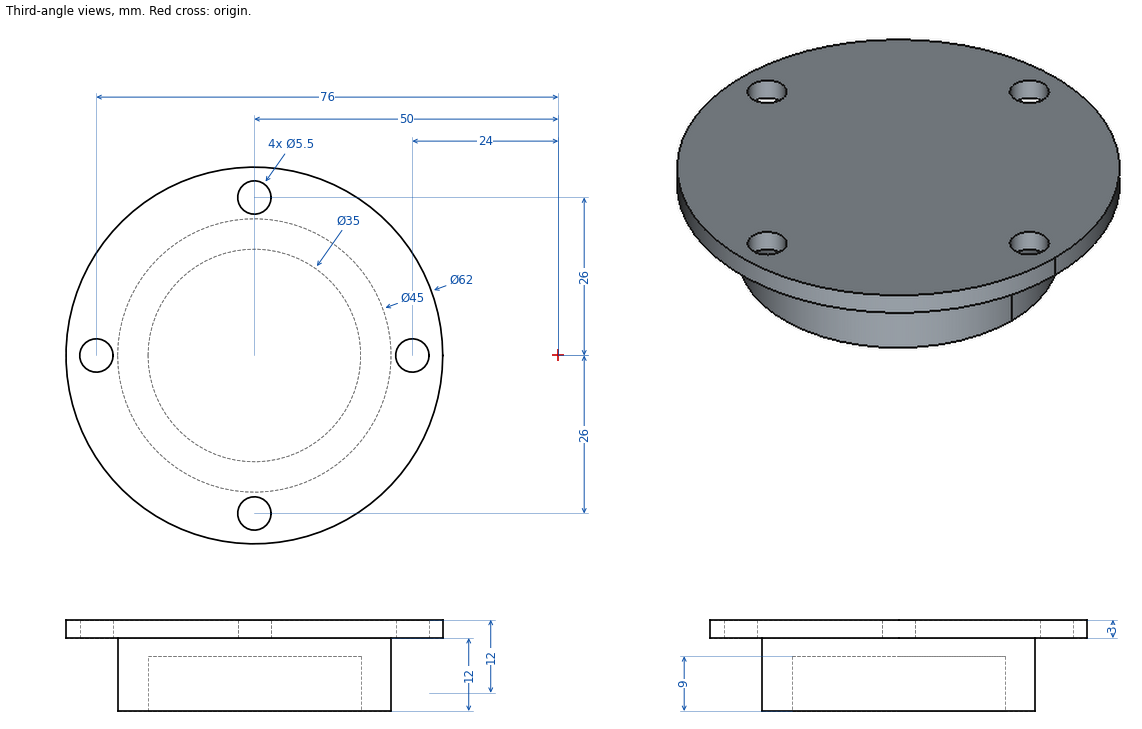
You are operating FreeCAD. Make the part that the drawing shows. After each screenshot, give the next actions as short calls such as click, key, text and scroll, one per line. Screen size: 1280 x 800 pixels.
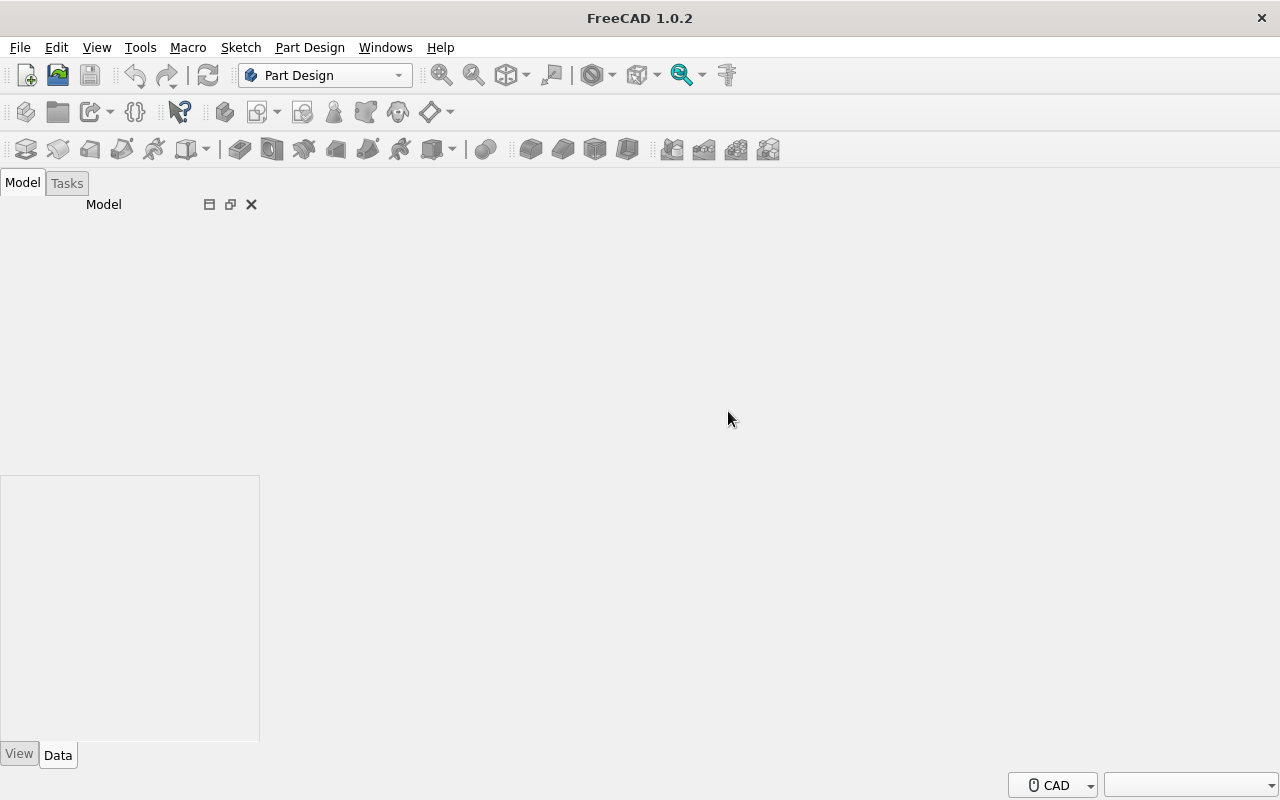
click(26, 76)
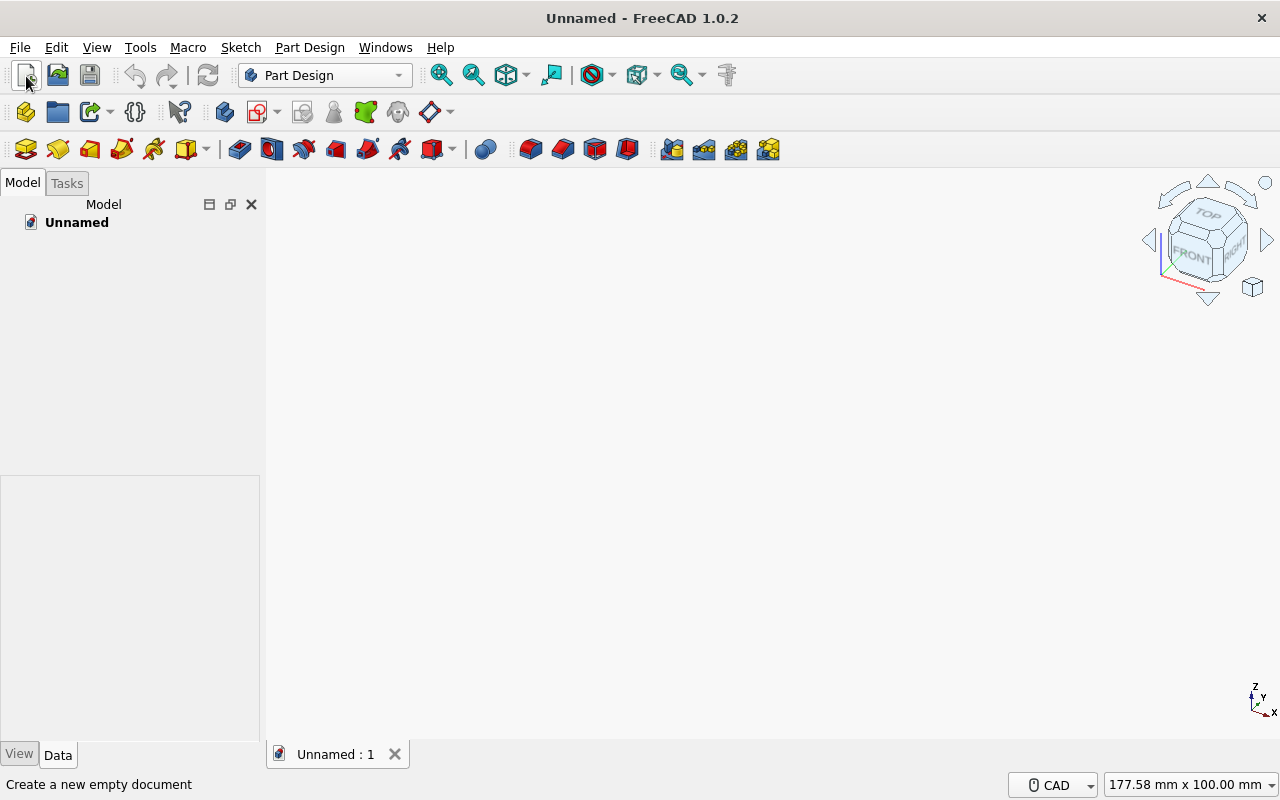
click(226, 112)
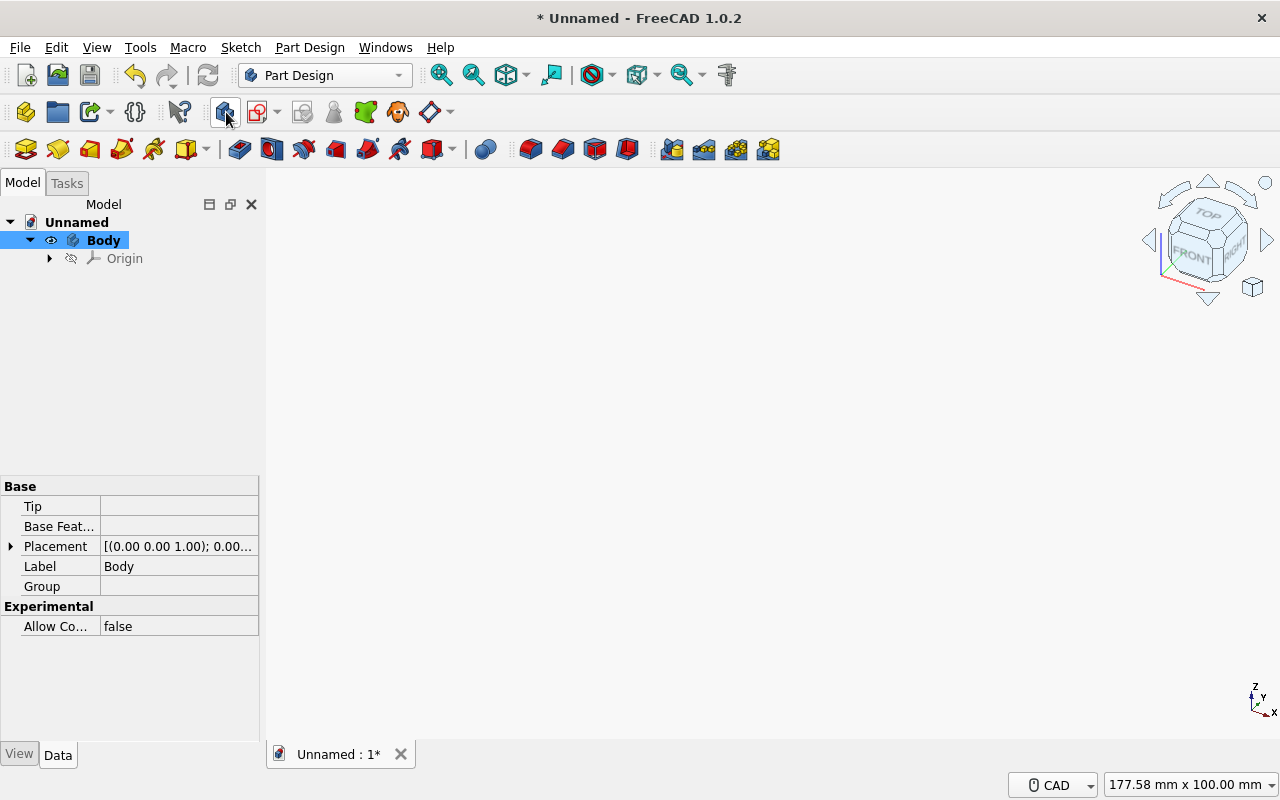
click(50, 258)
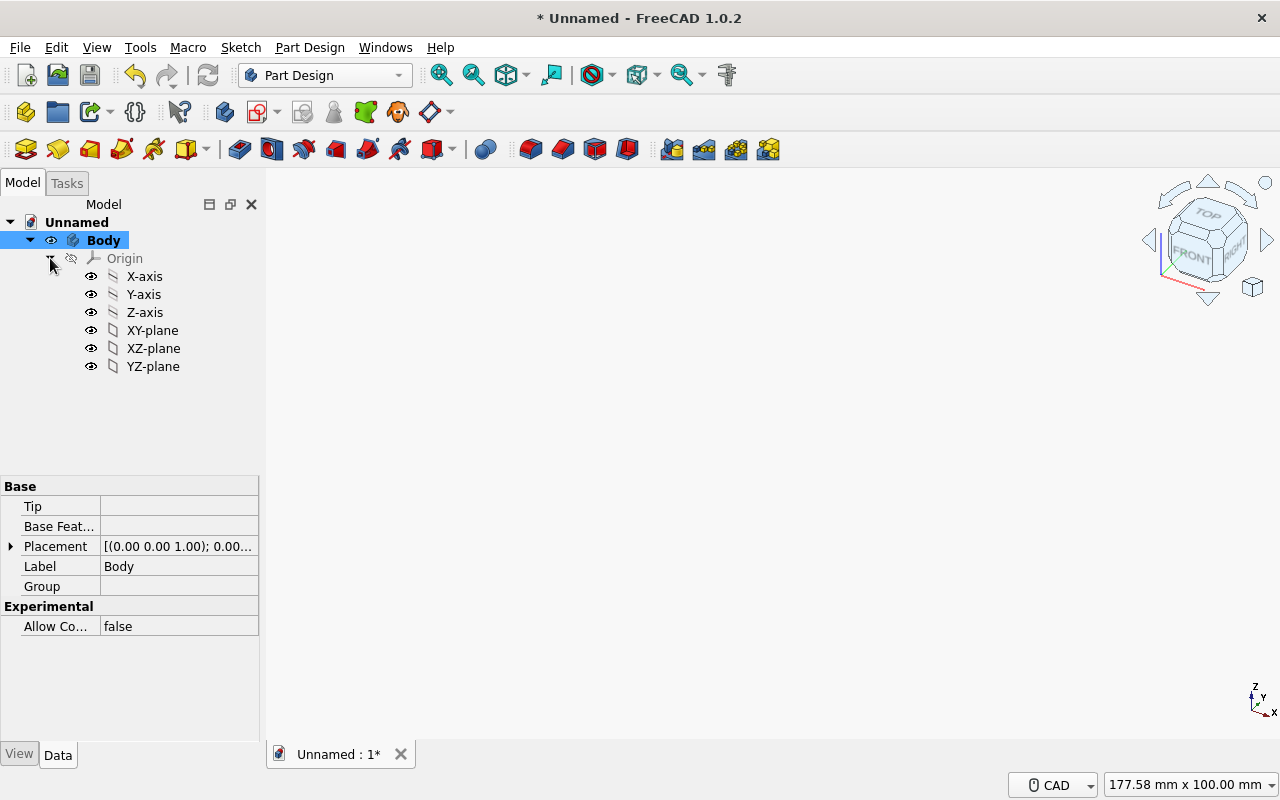
click(136, 330)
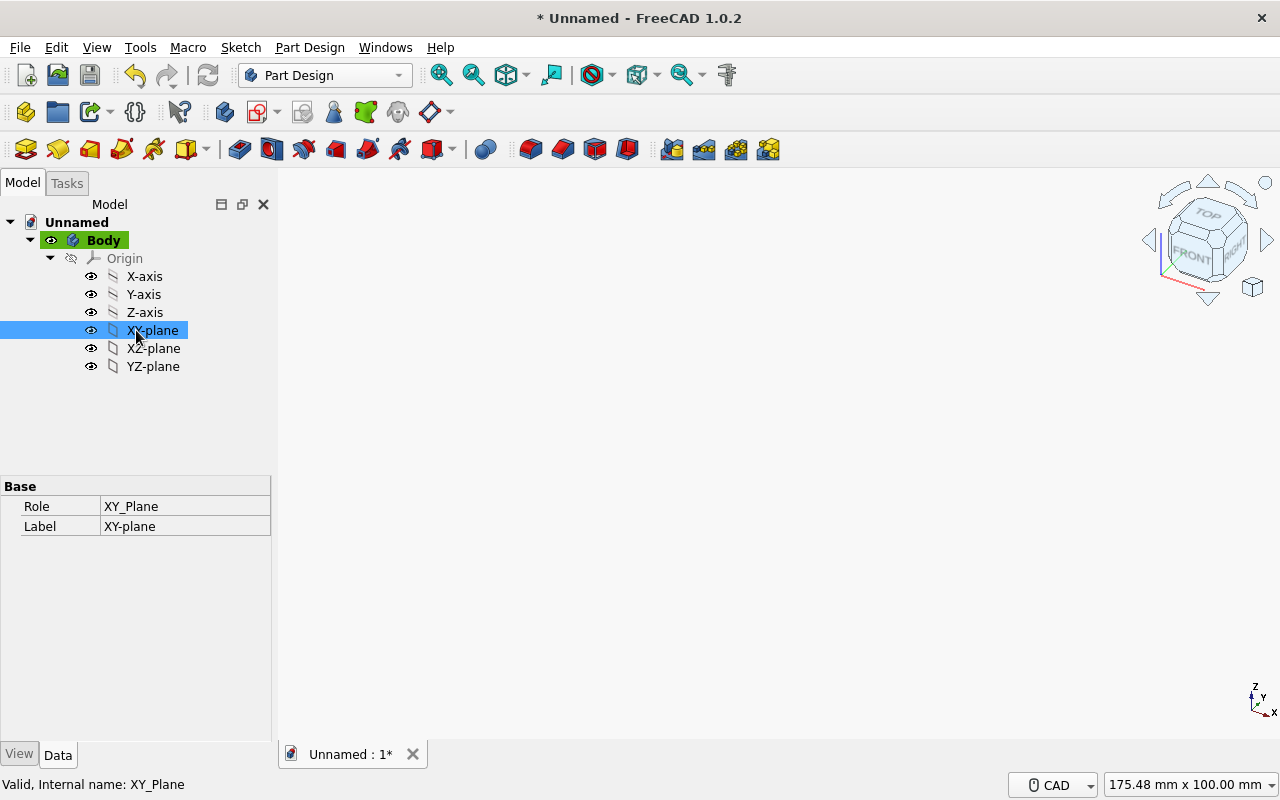
click(430, 112)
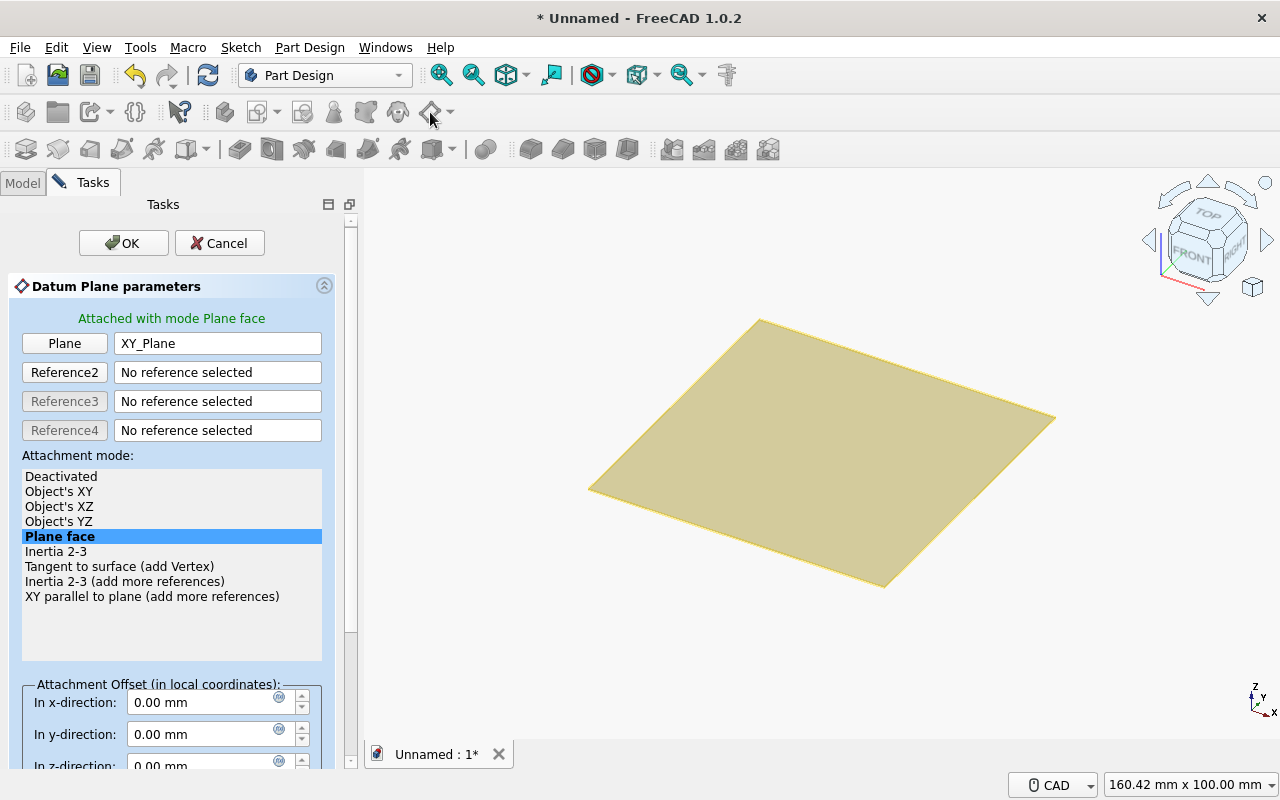
scroll(351, 491, down, 2)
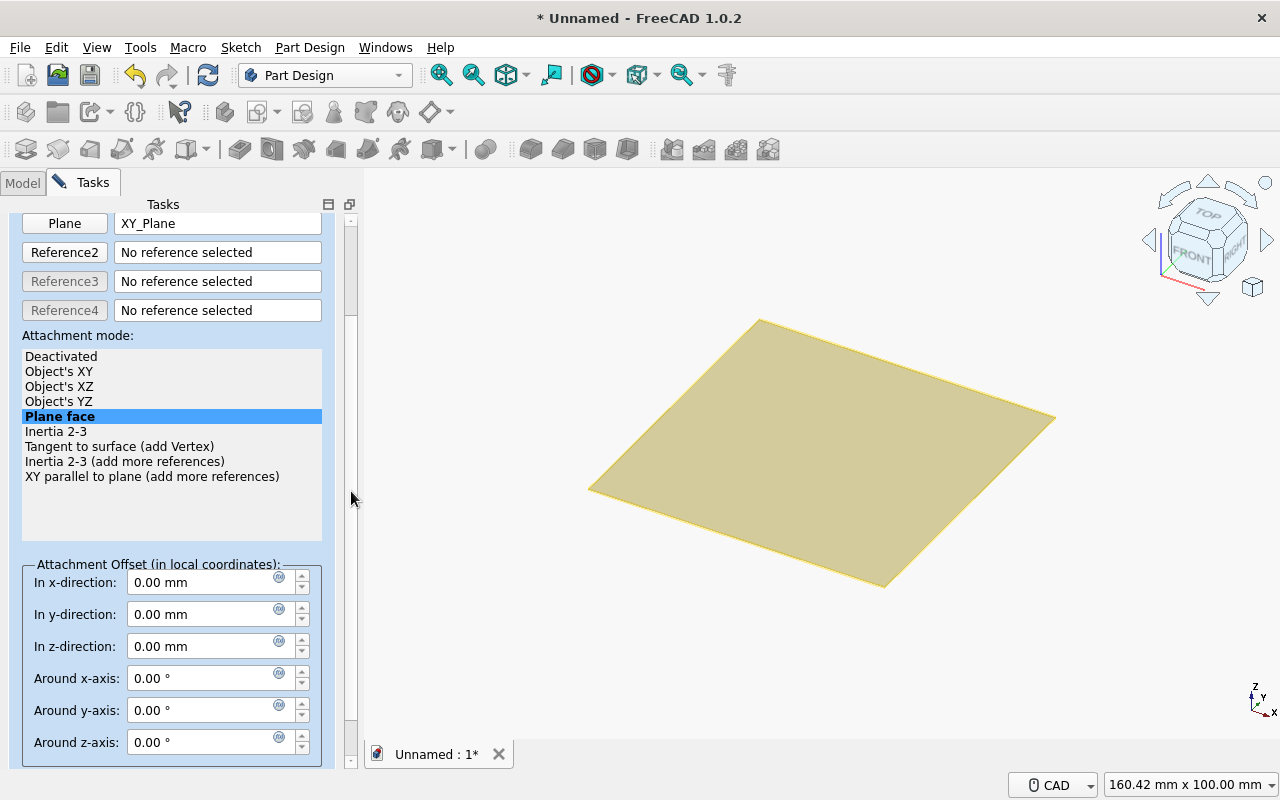
triple_click(210, 646)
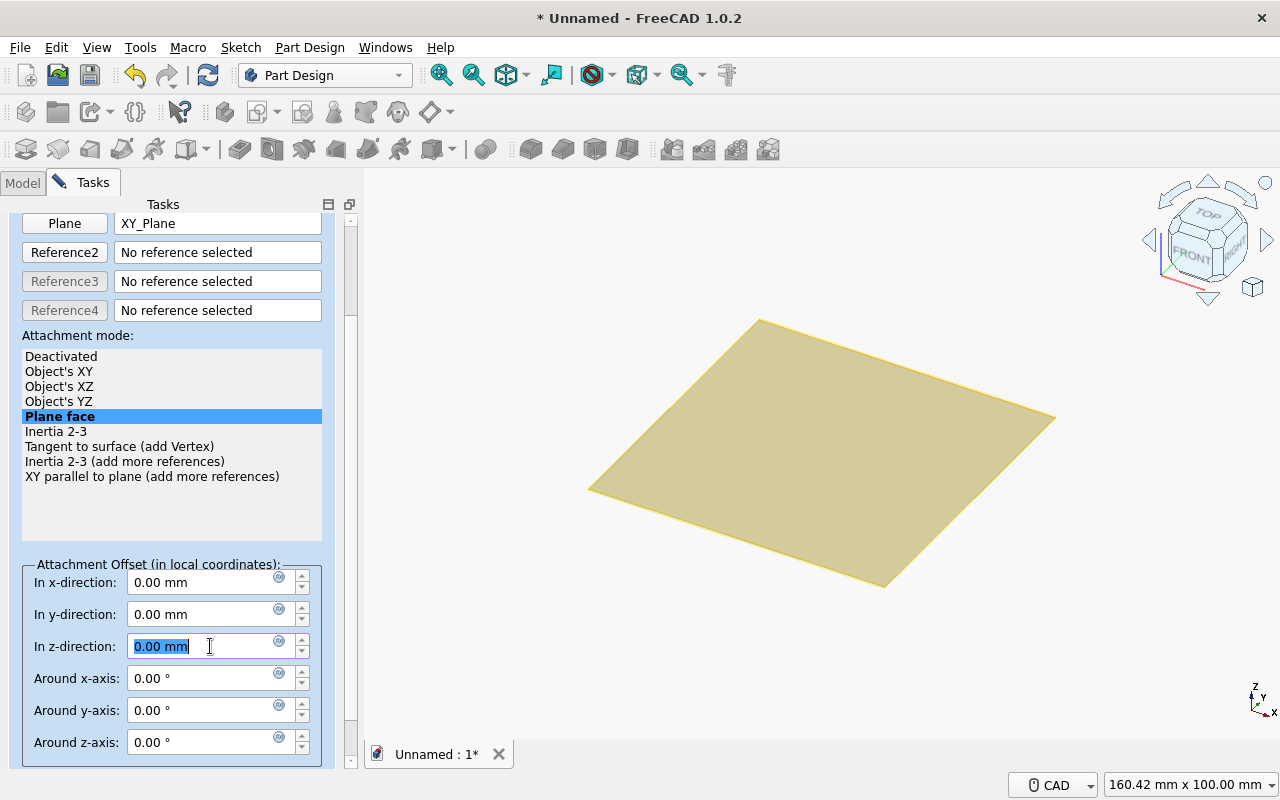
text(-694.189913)
key(Tab)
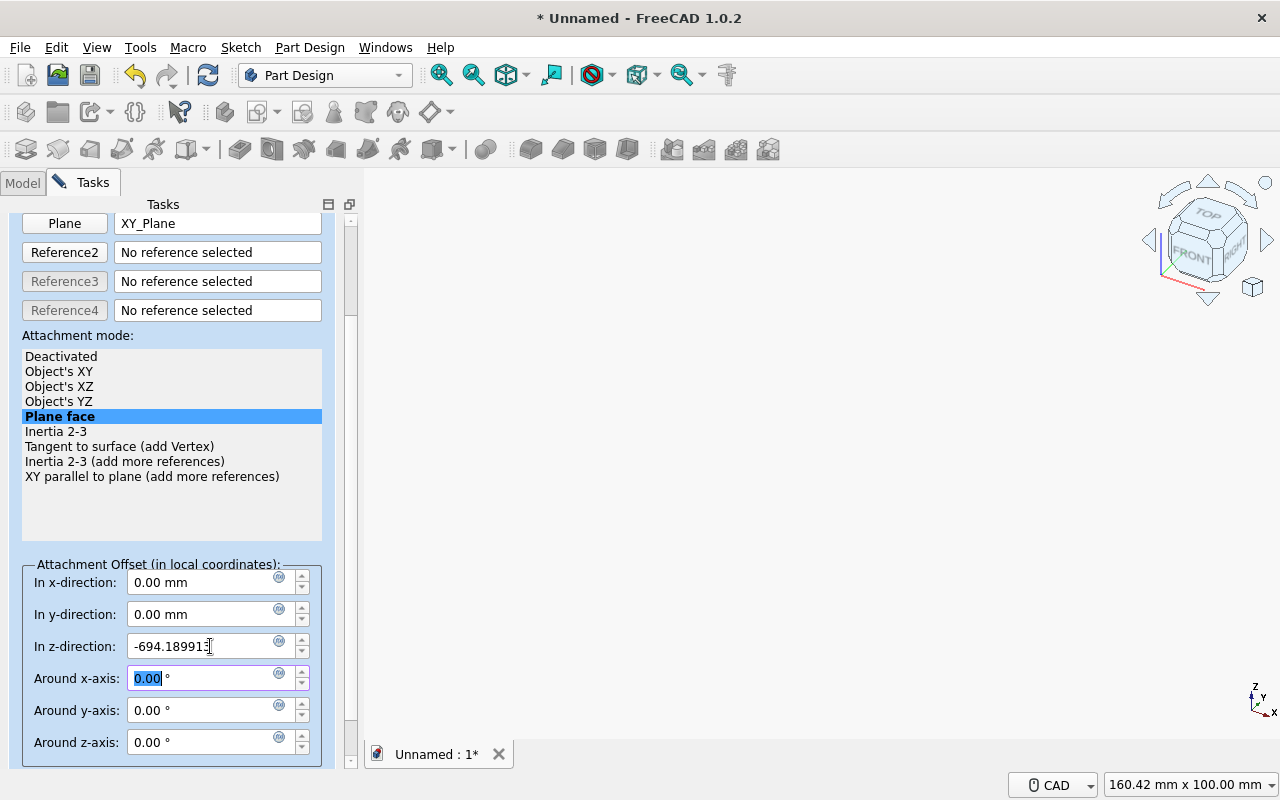
scroll(351, 491, up, 3)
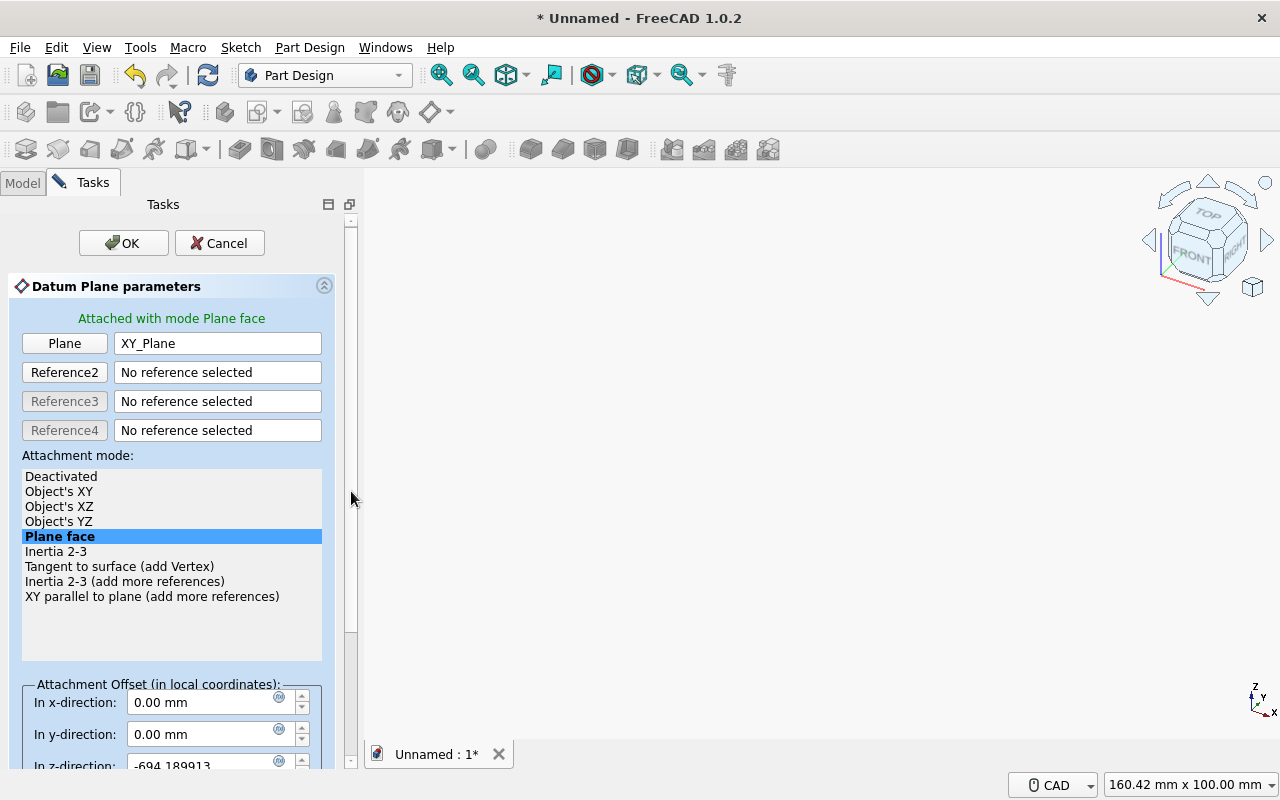
click(124, 243)